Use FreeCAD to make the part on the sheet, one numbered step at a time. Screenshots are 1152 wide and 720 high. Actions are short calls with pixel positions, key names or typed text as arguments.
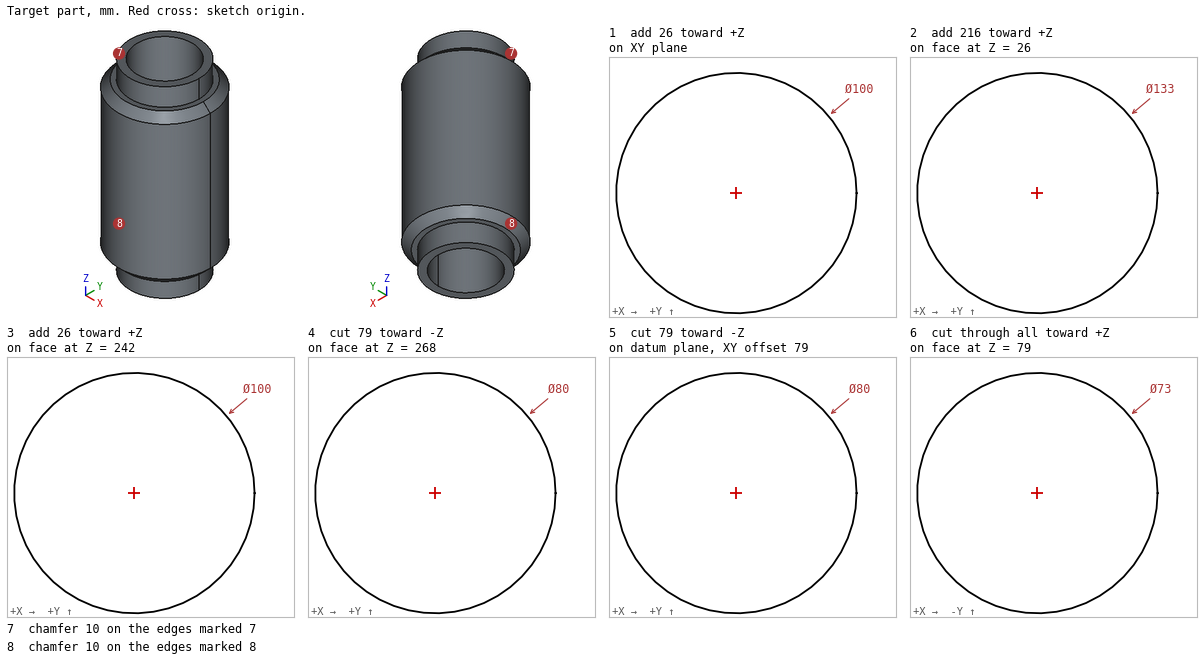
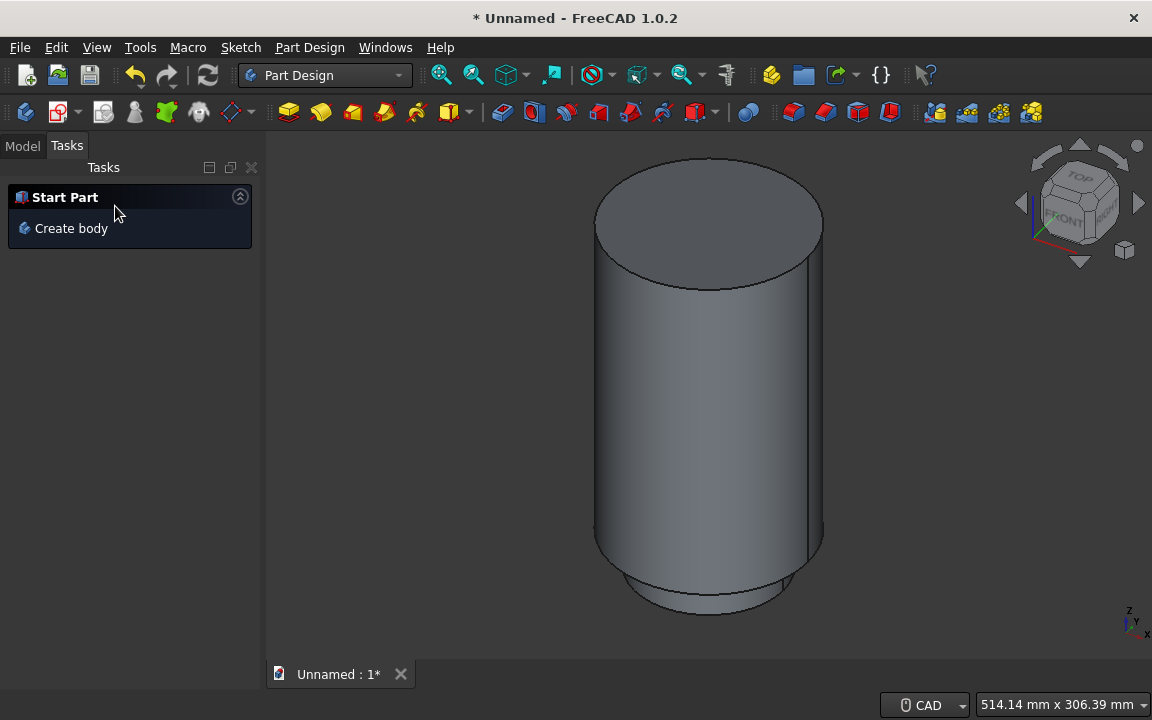
click(709, 223)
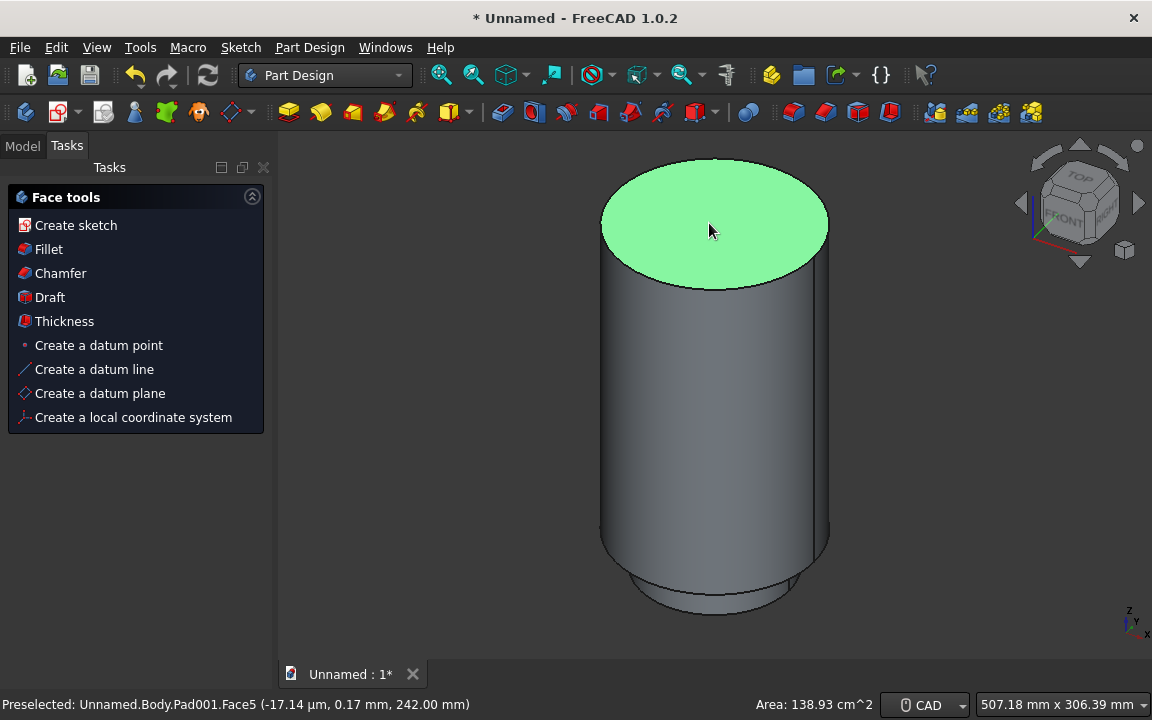
click(58, 112)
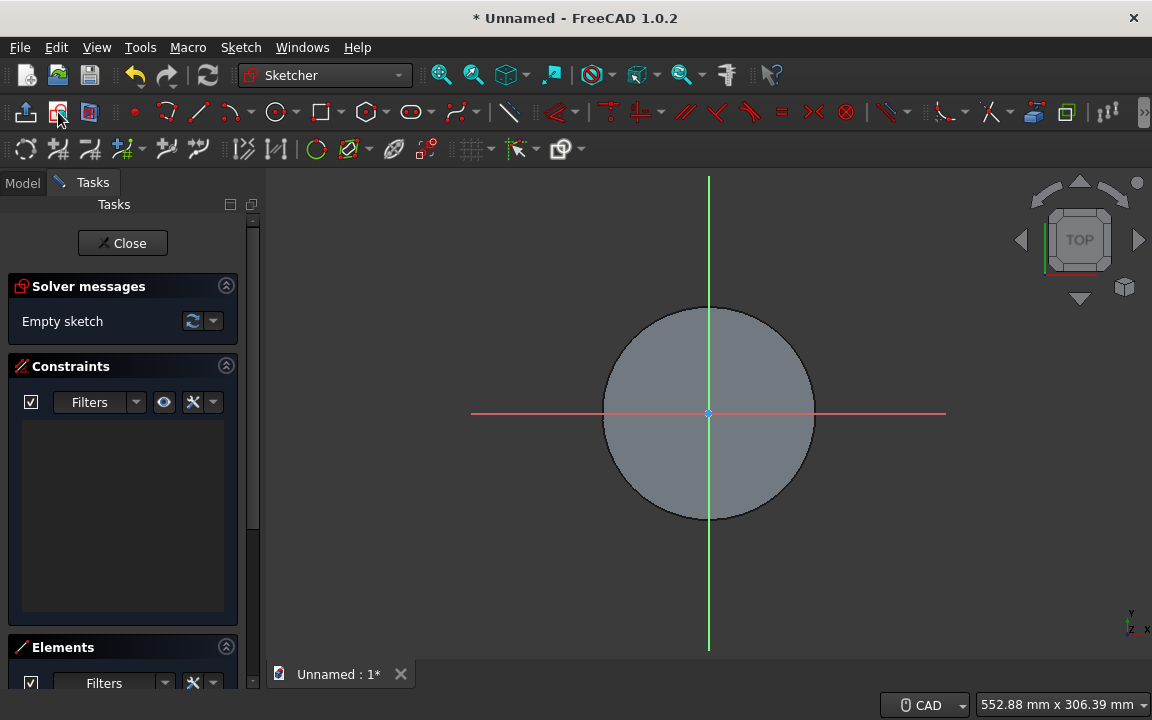
scroll(792, 414, up, 3)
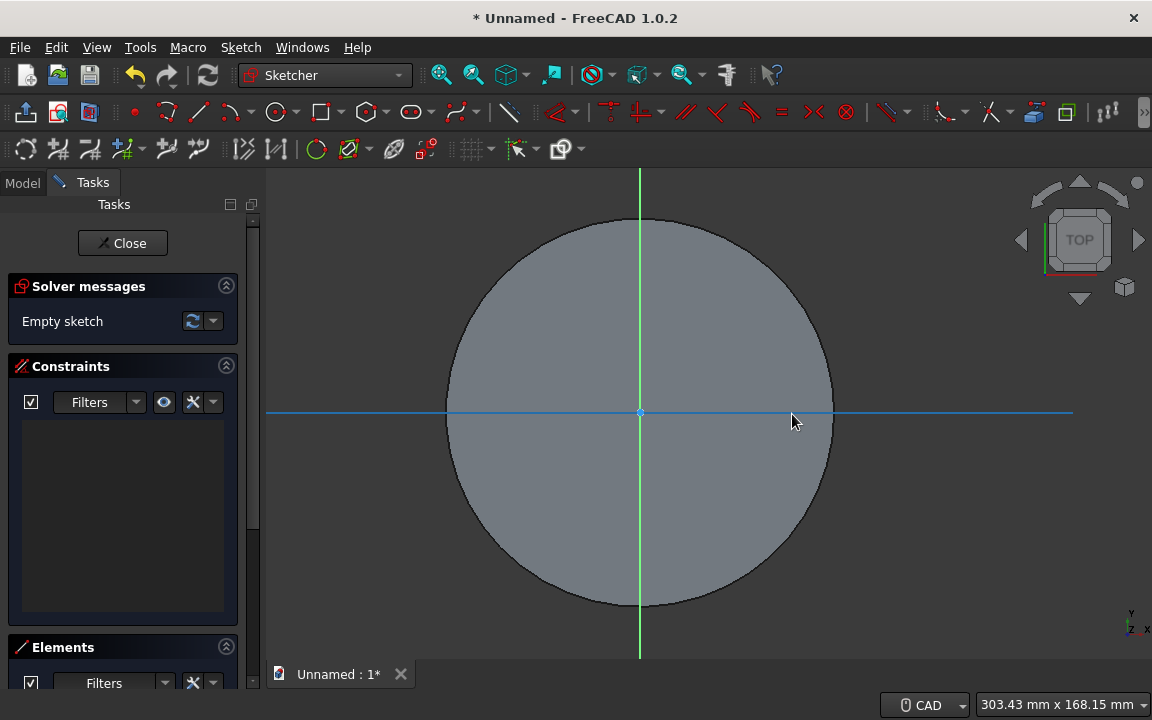
key(g)
key(c)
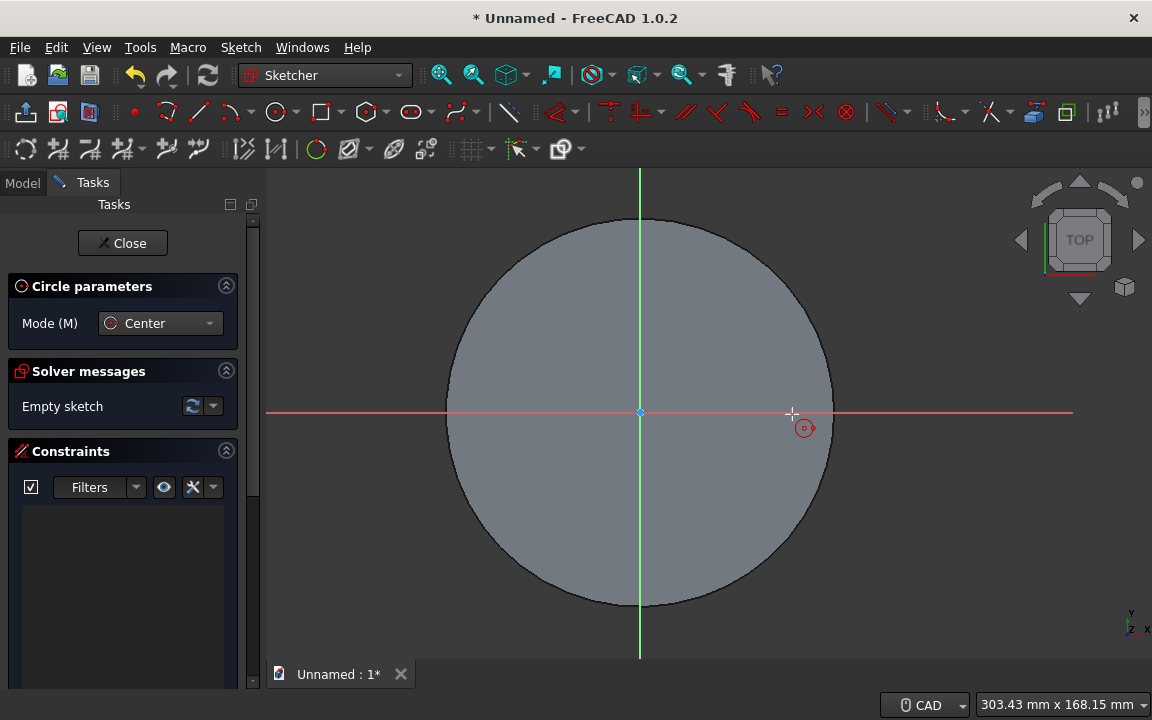
click(640, 413)
move(743, 309)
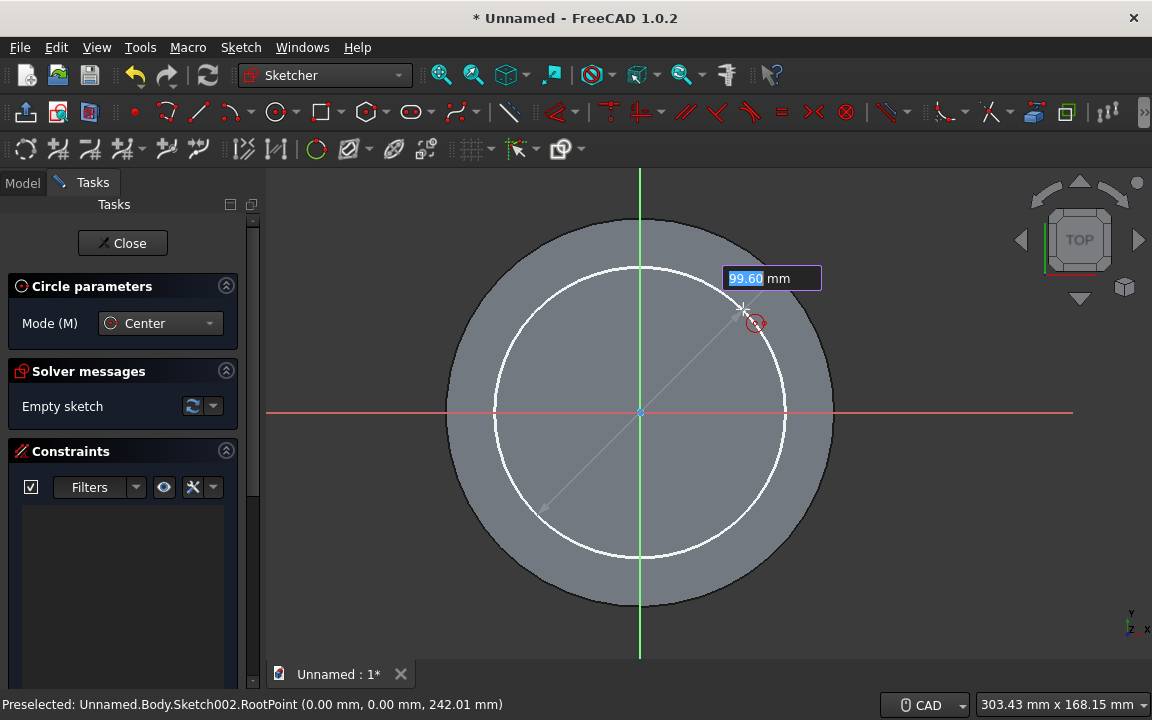
text(100)
key(Return)
key(Escape)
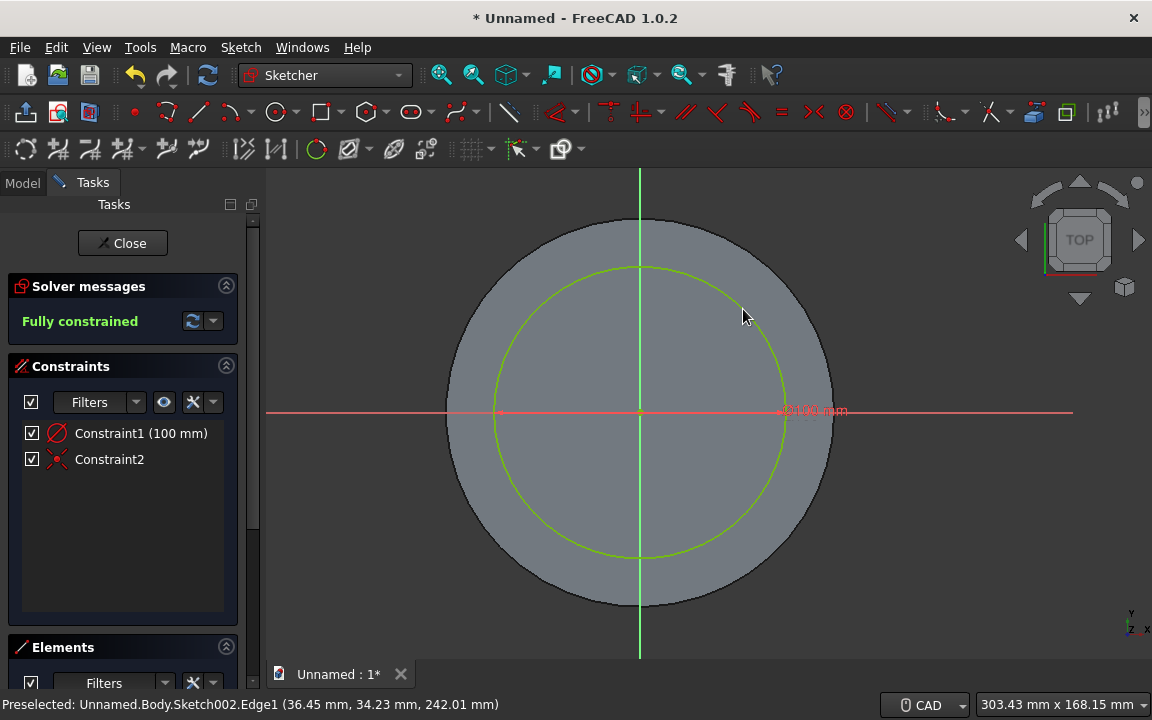
click(123, 243)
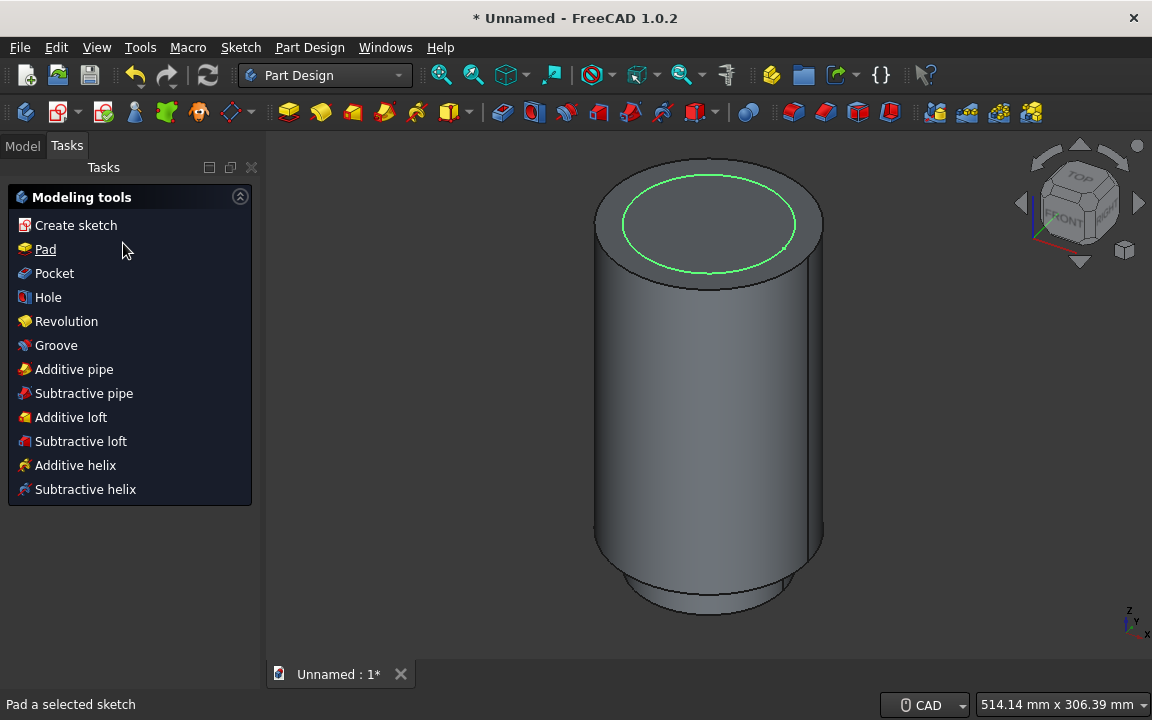
click(290, 112)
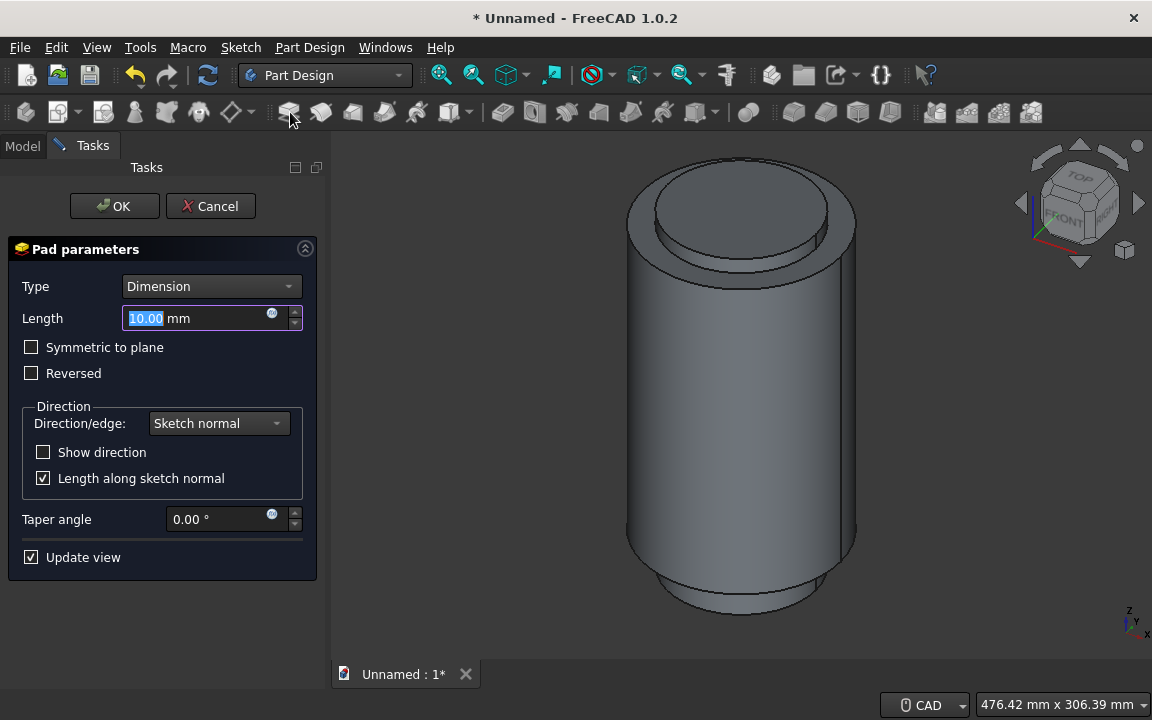
text(26)
key(Tab)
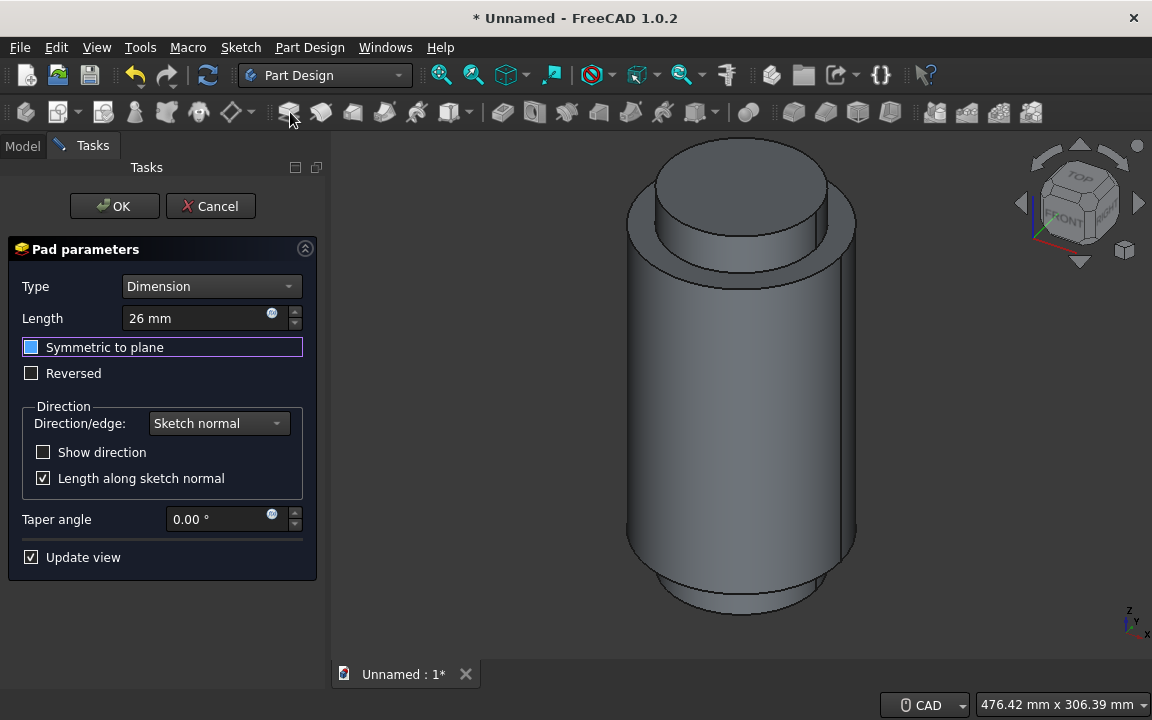
click(115, 206)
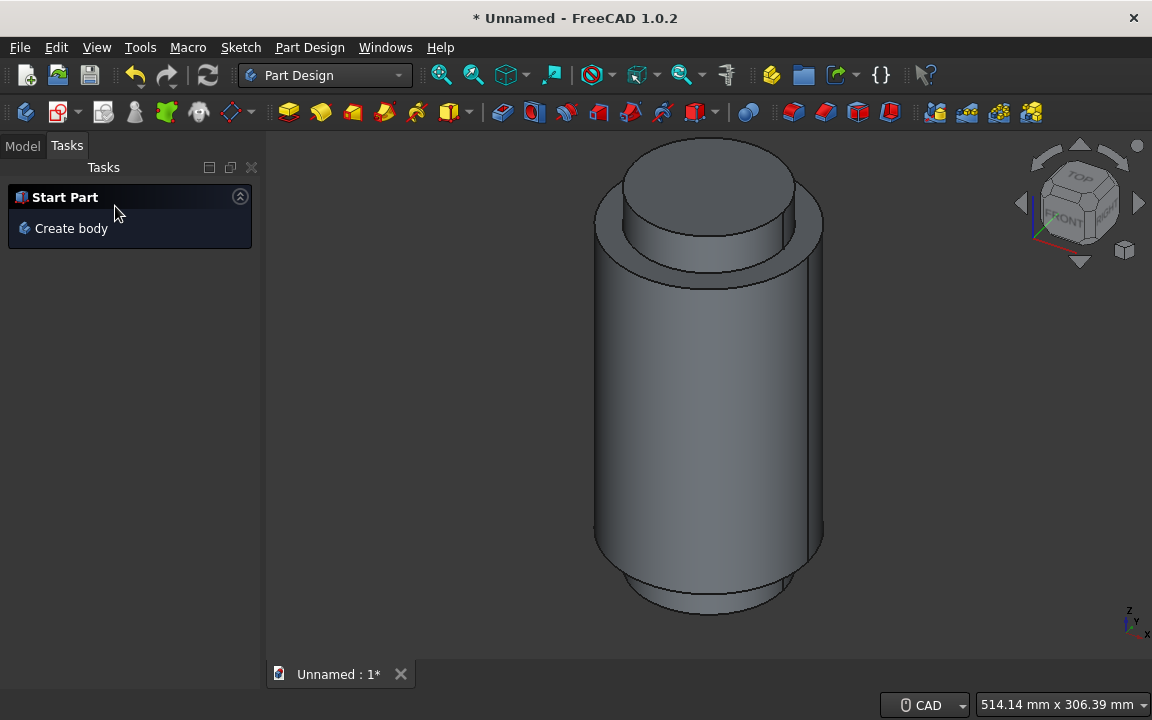
key(v)
key(f)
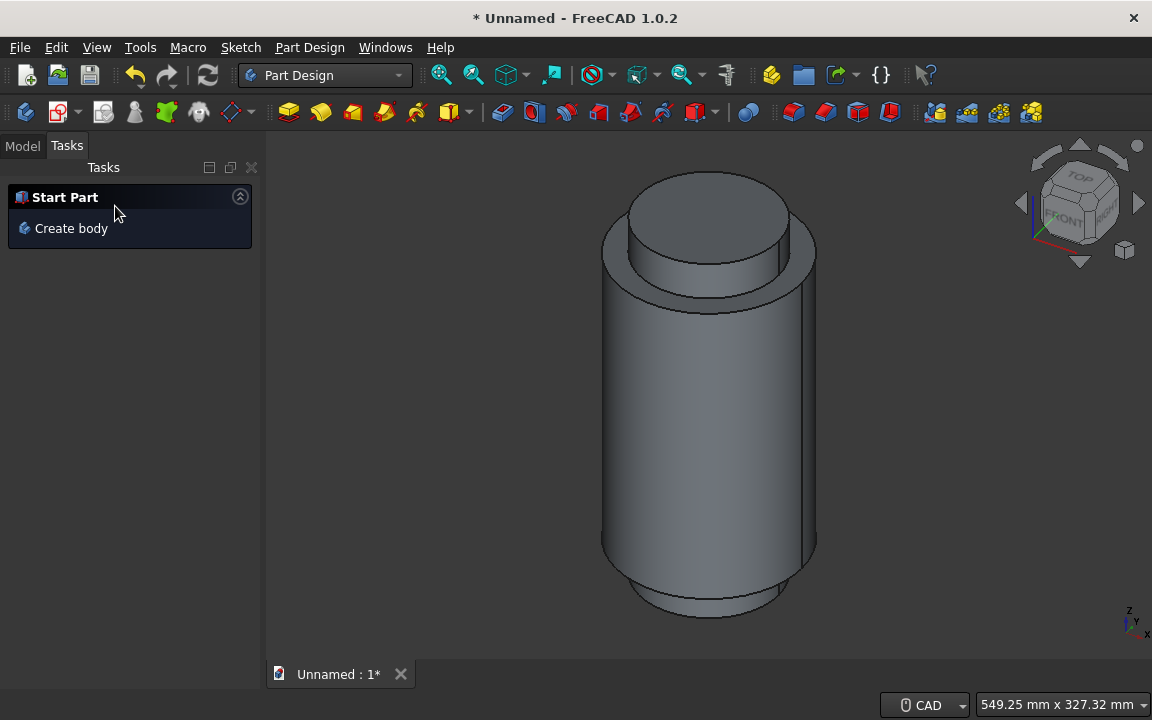
click(709, 217)